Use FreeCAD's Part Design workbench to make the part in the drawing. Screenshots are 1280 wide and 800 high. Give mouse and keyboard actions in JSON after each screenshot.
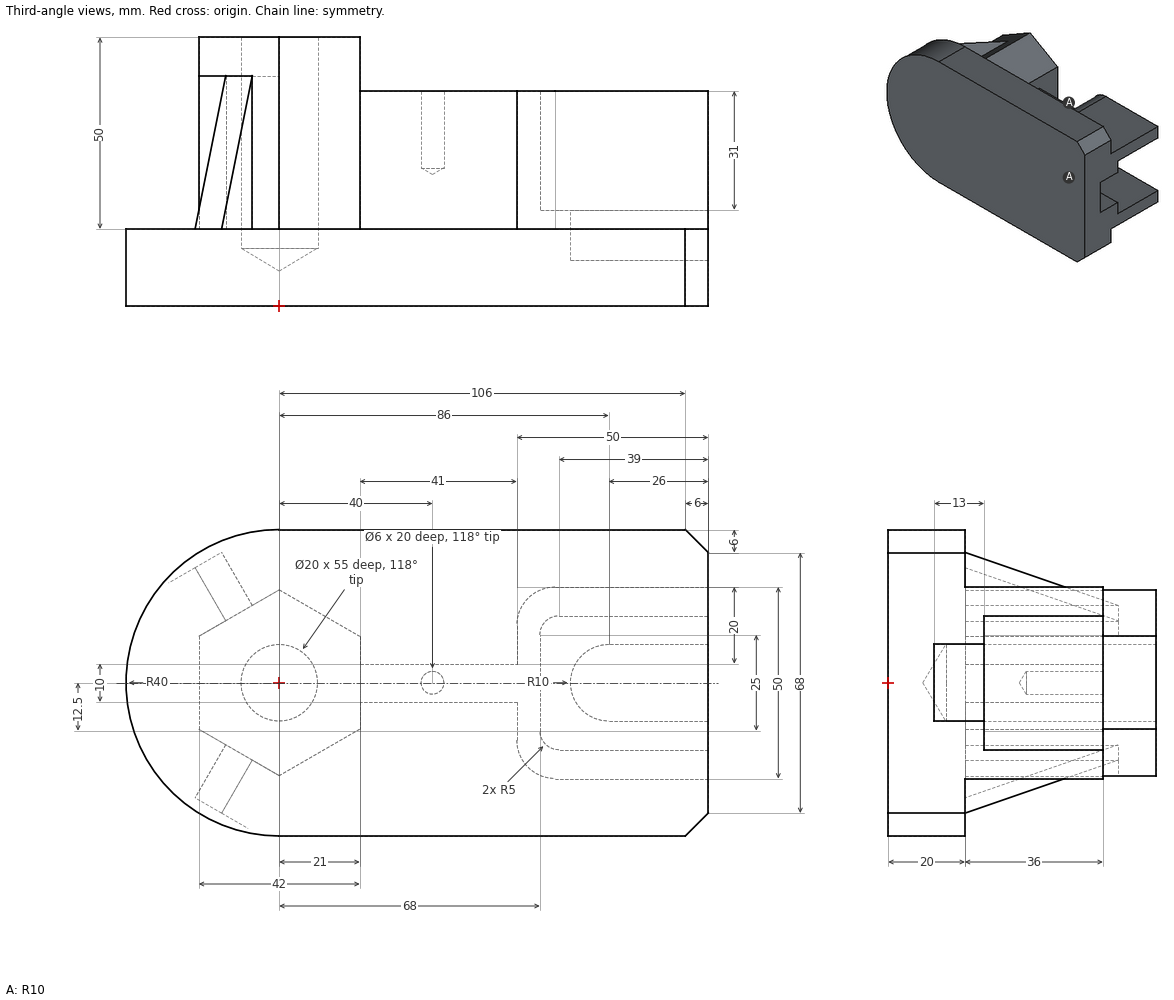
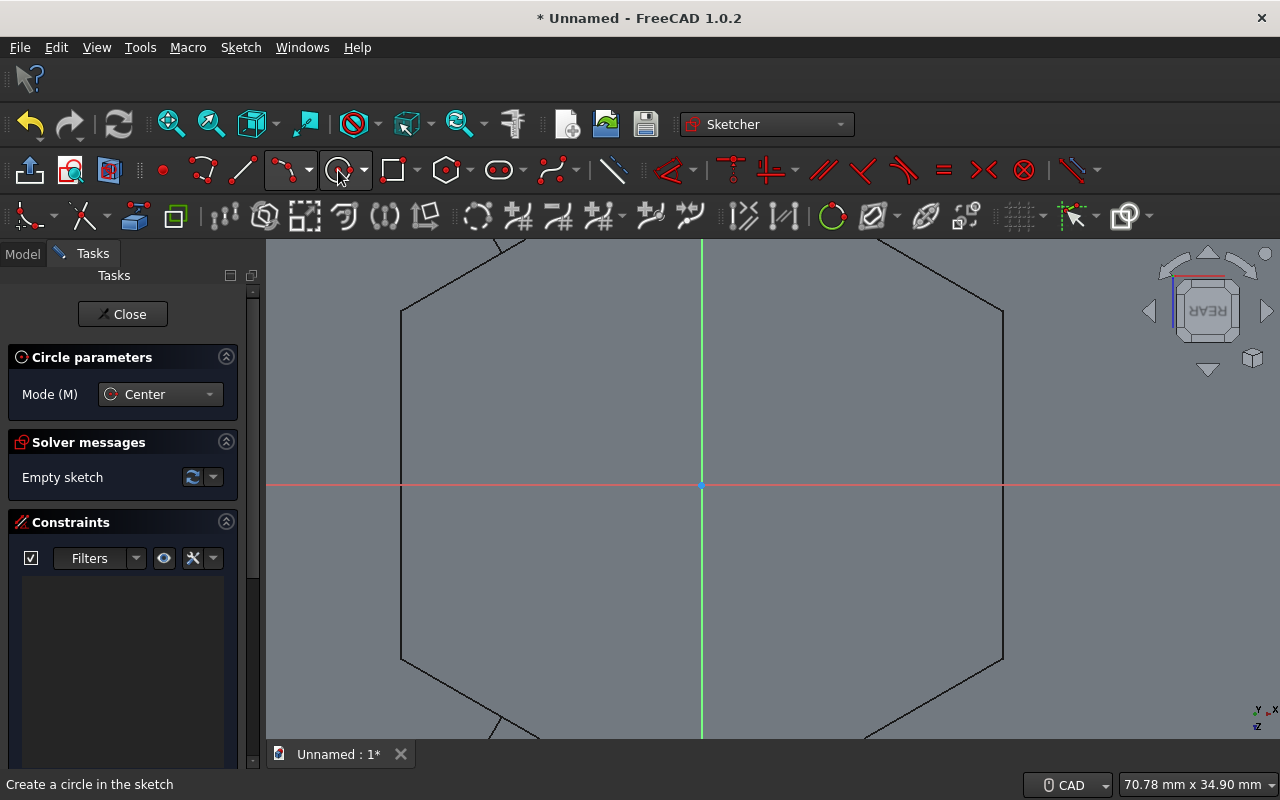
{"action": "left_click", "coordinate": [702, 485]}
{"action": "mouse_move", "coordinate": [803, 384]}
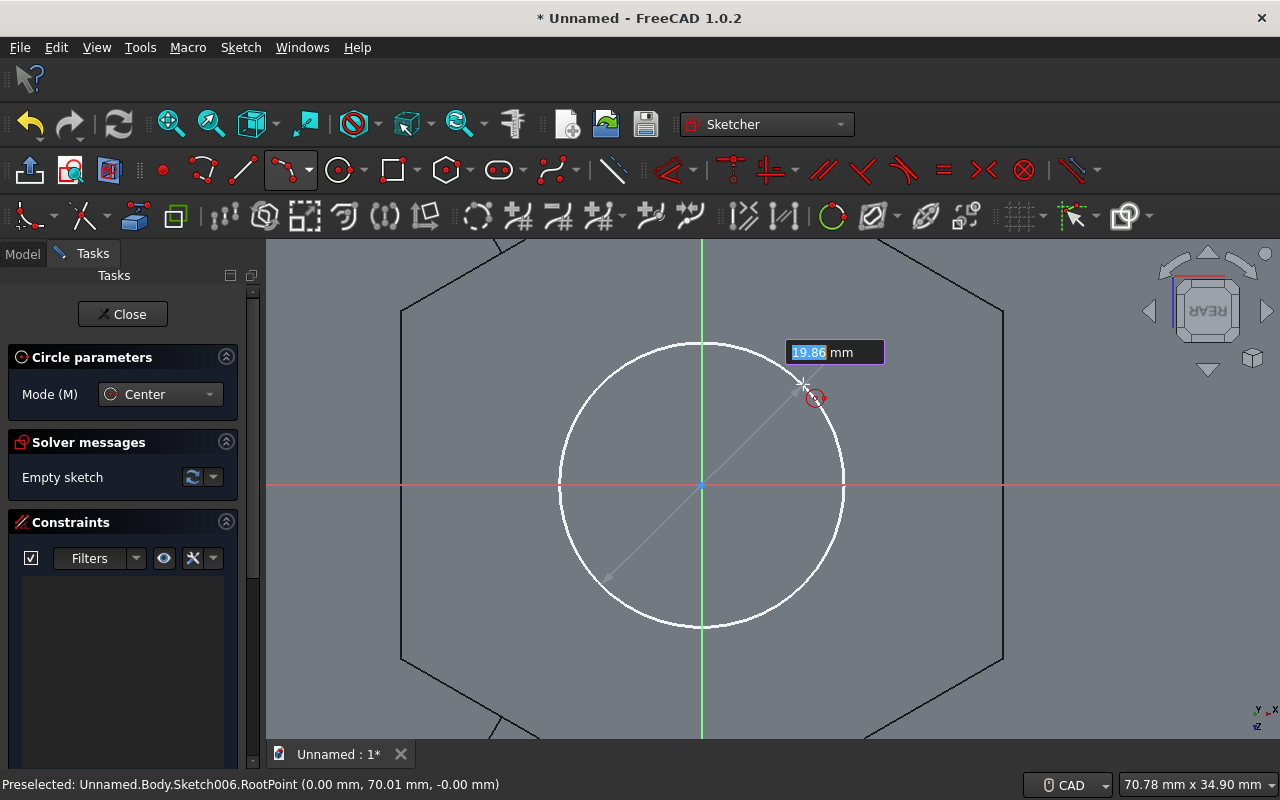
{"action": "type", "text": "20"}
{"action": "key", "text": "Return"}
{"action": "key", "text": "Escape"}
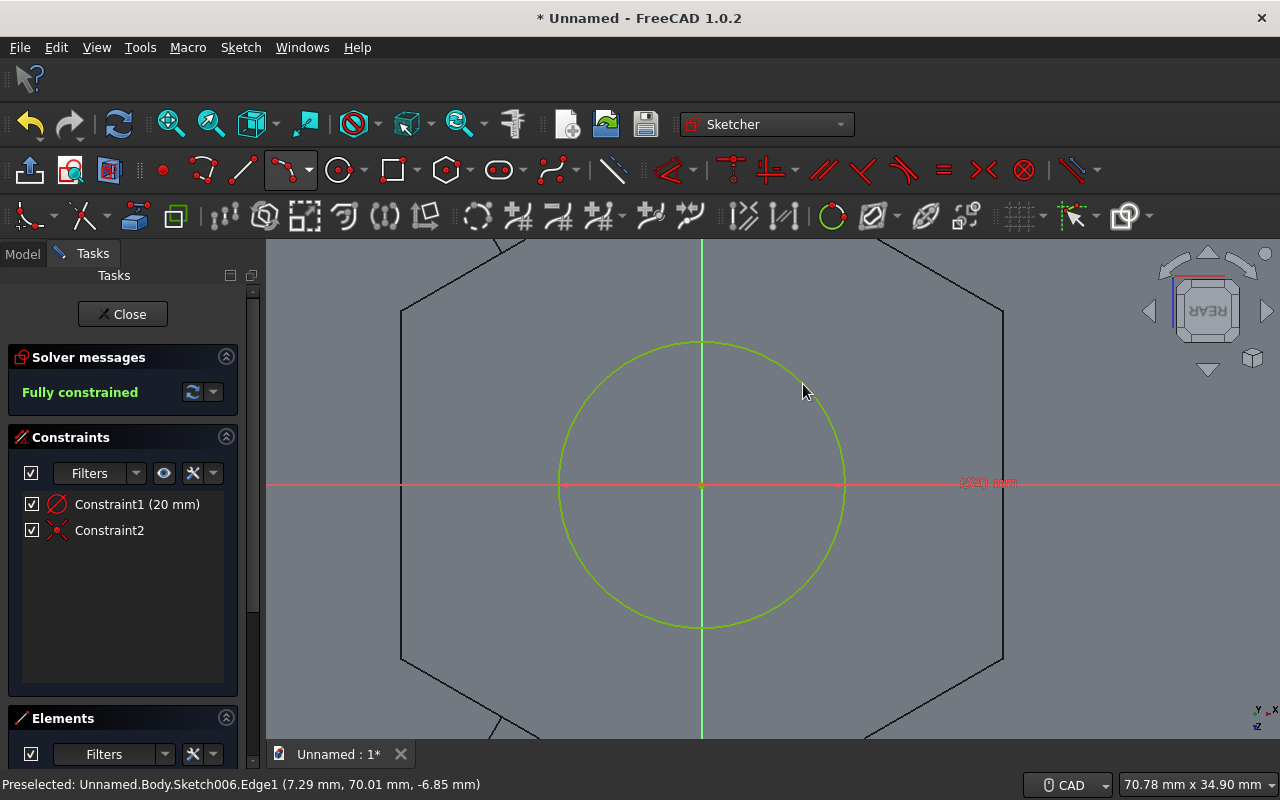
{"action": "left_click", "coordinate": [123, 314]}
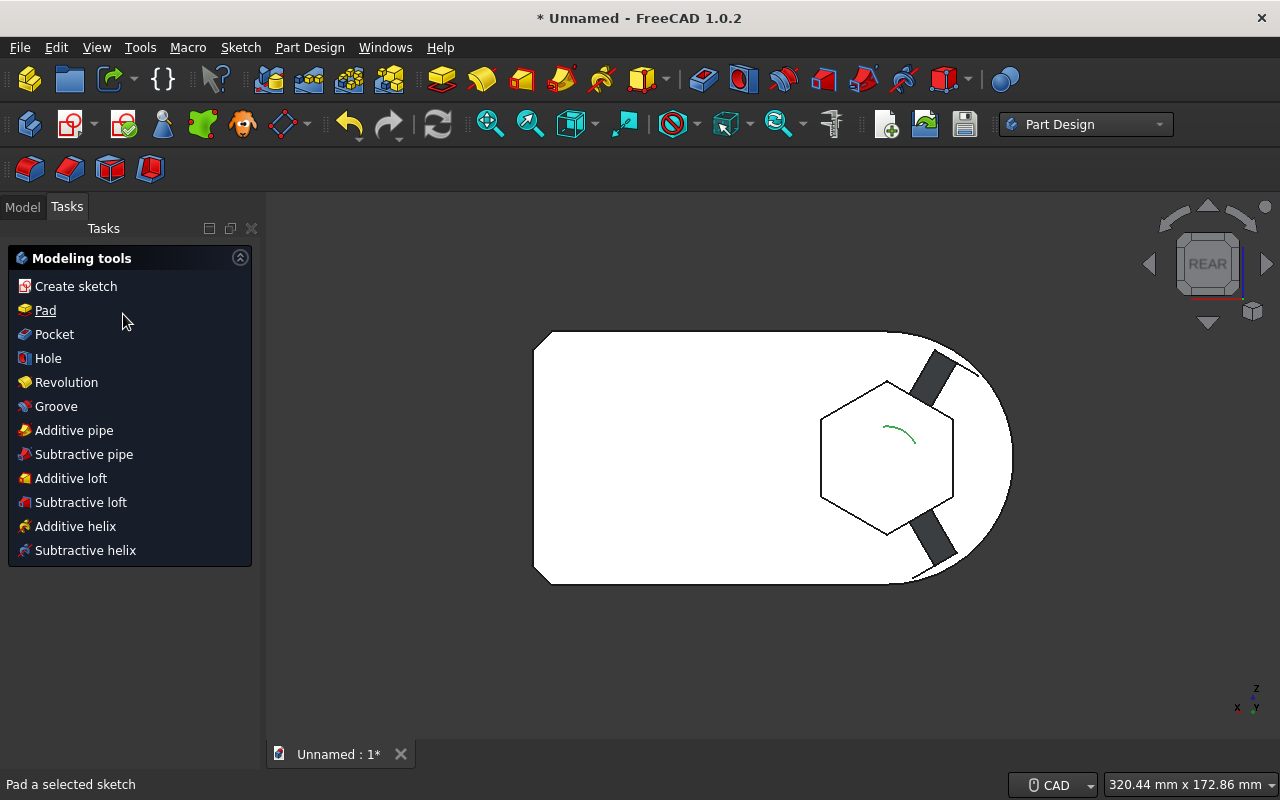
{"action": "left_click", "coordinate": [744, 80]}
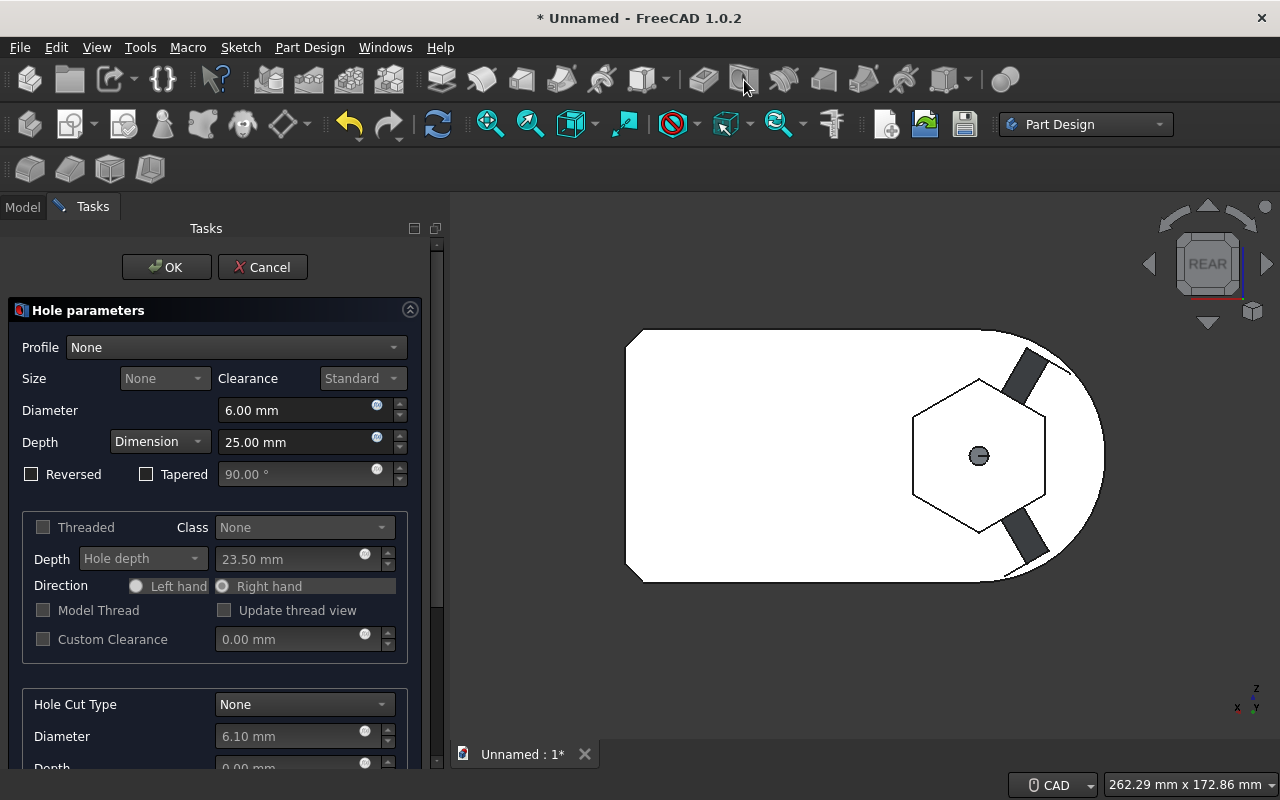
{"action": "triple_click", "coordinate": [305, 410]}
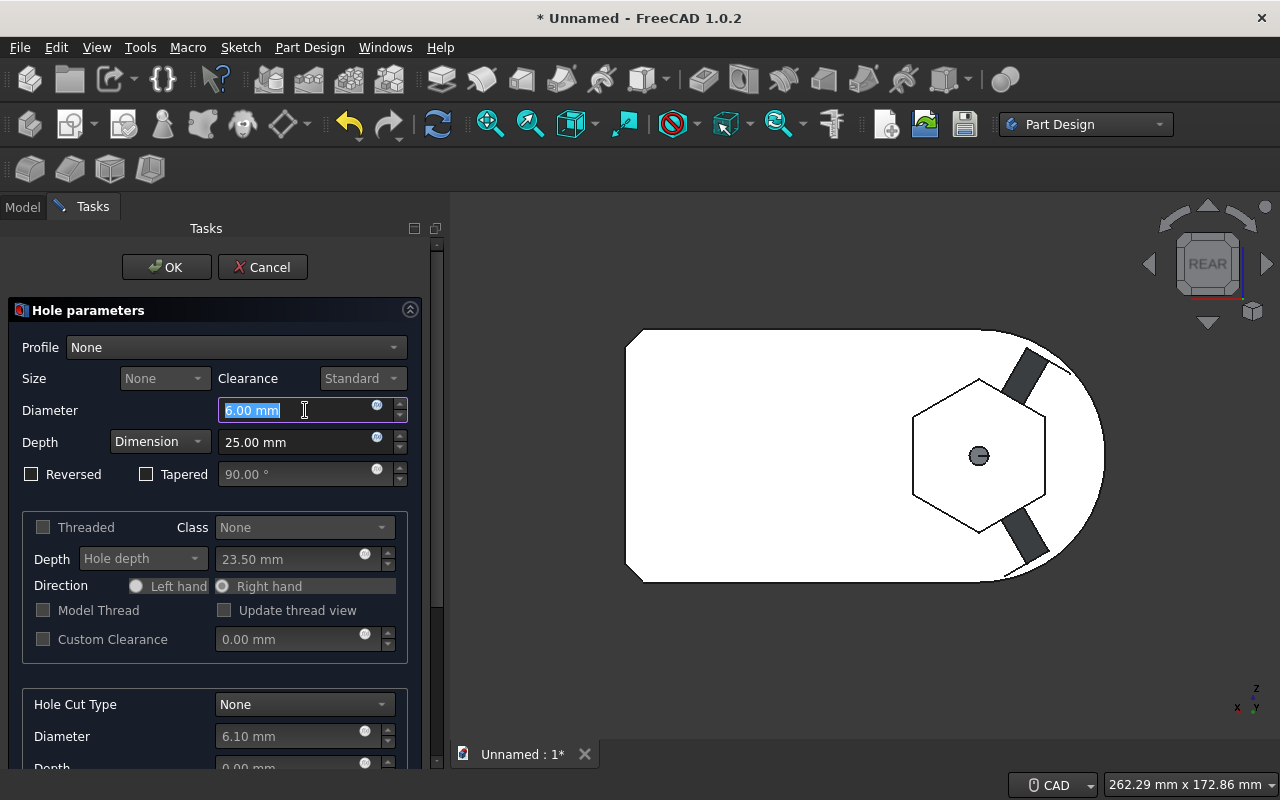
{"action": "type", "text": "20"}
{"action": "key", "text": "Tab"}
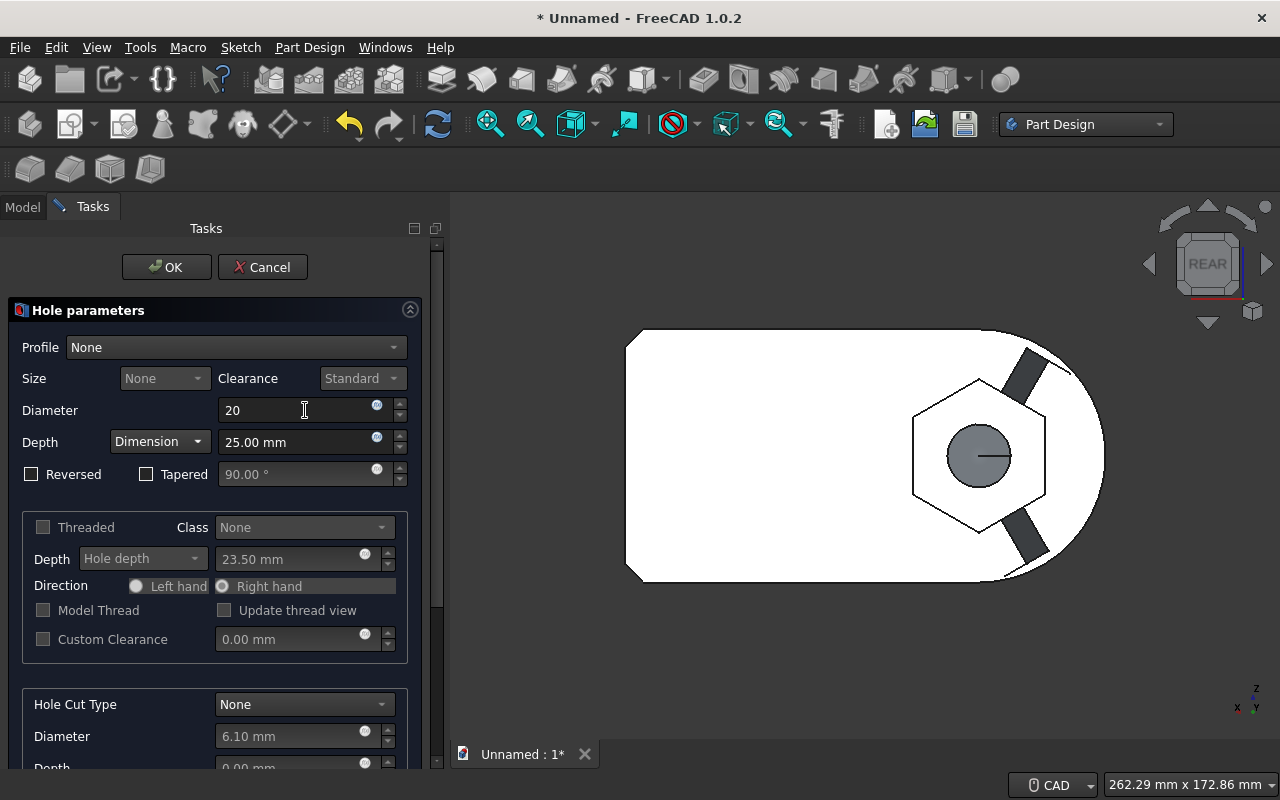
{"action": "triple_click", "coordinate": [305, 442]}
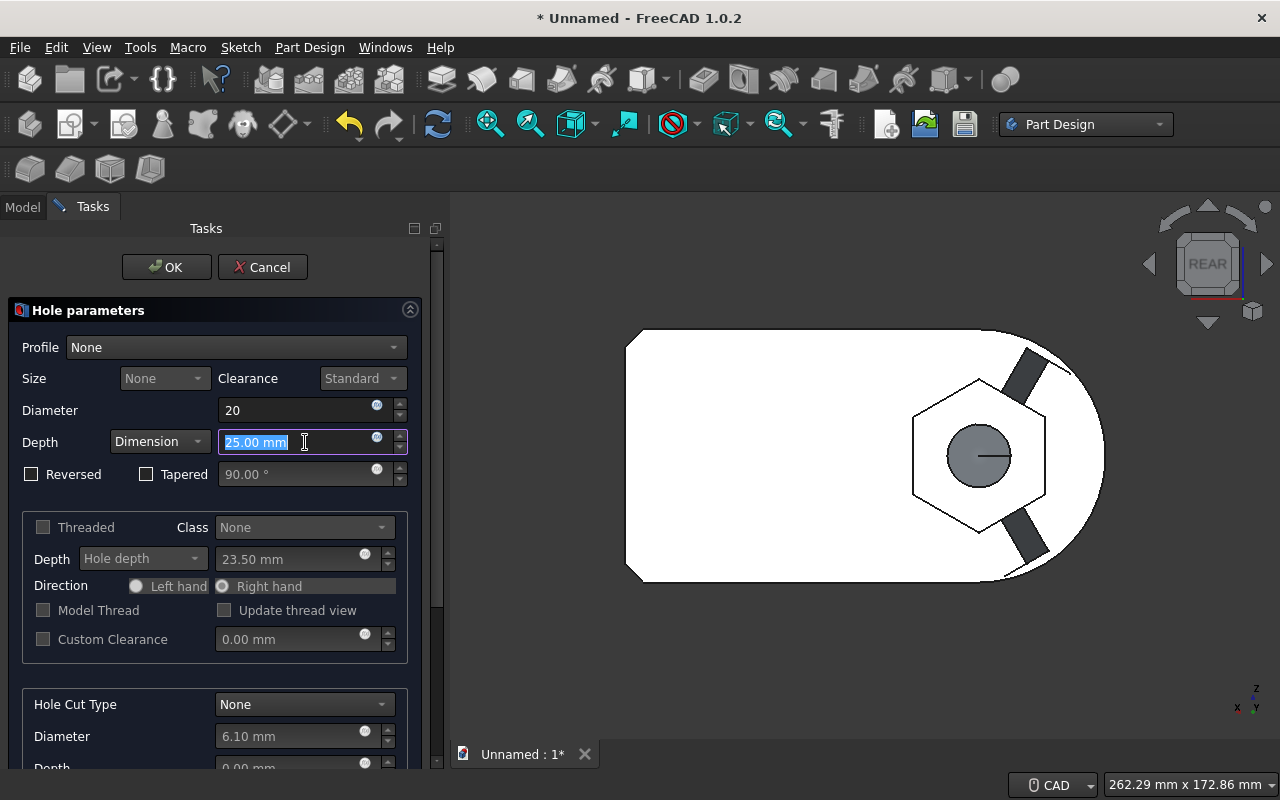
{"action": "type", "text": "55"}
{"action": "key", "text": "Tab"}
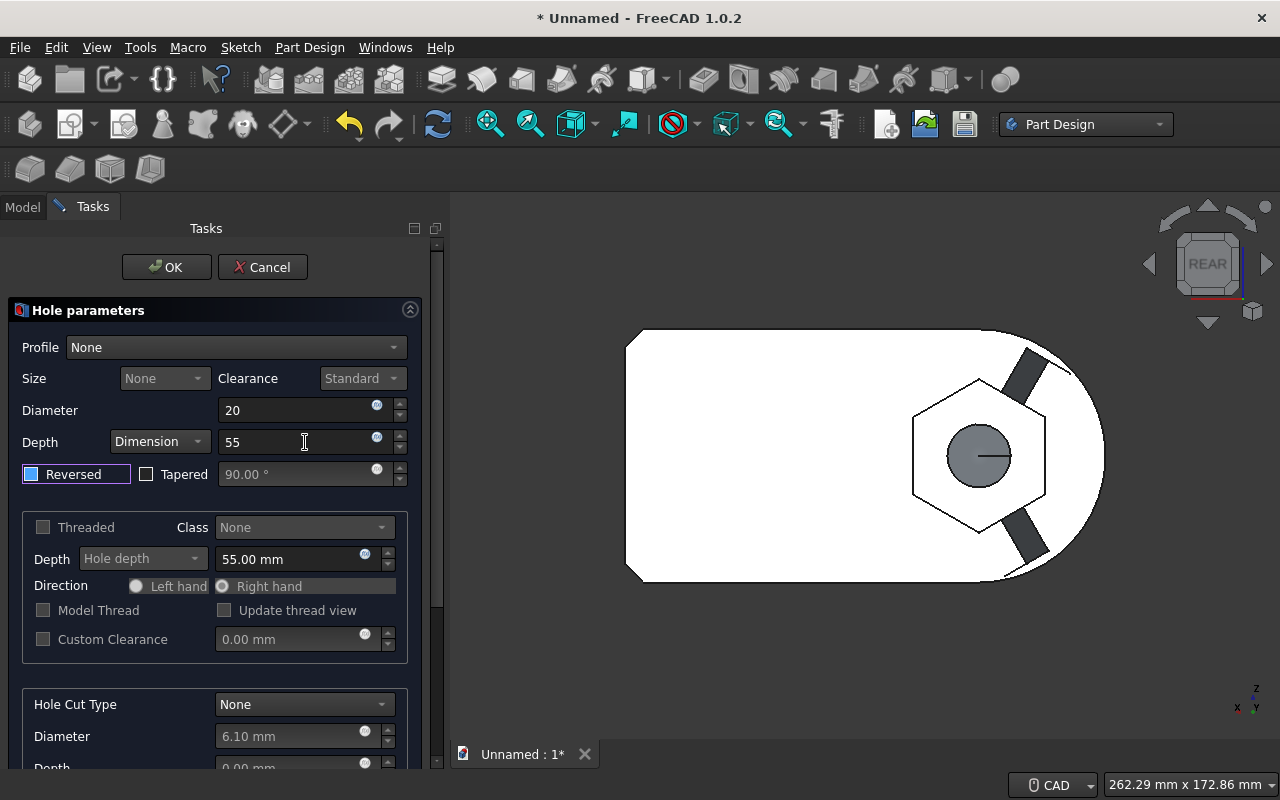
{"action": "left_click", "coordinate": [167, 267]}